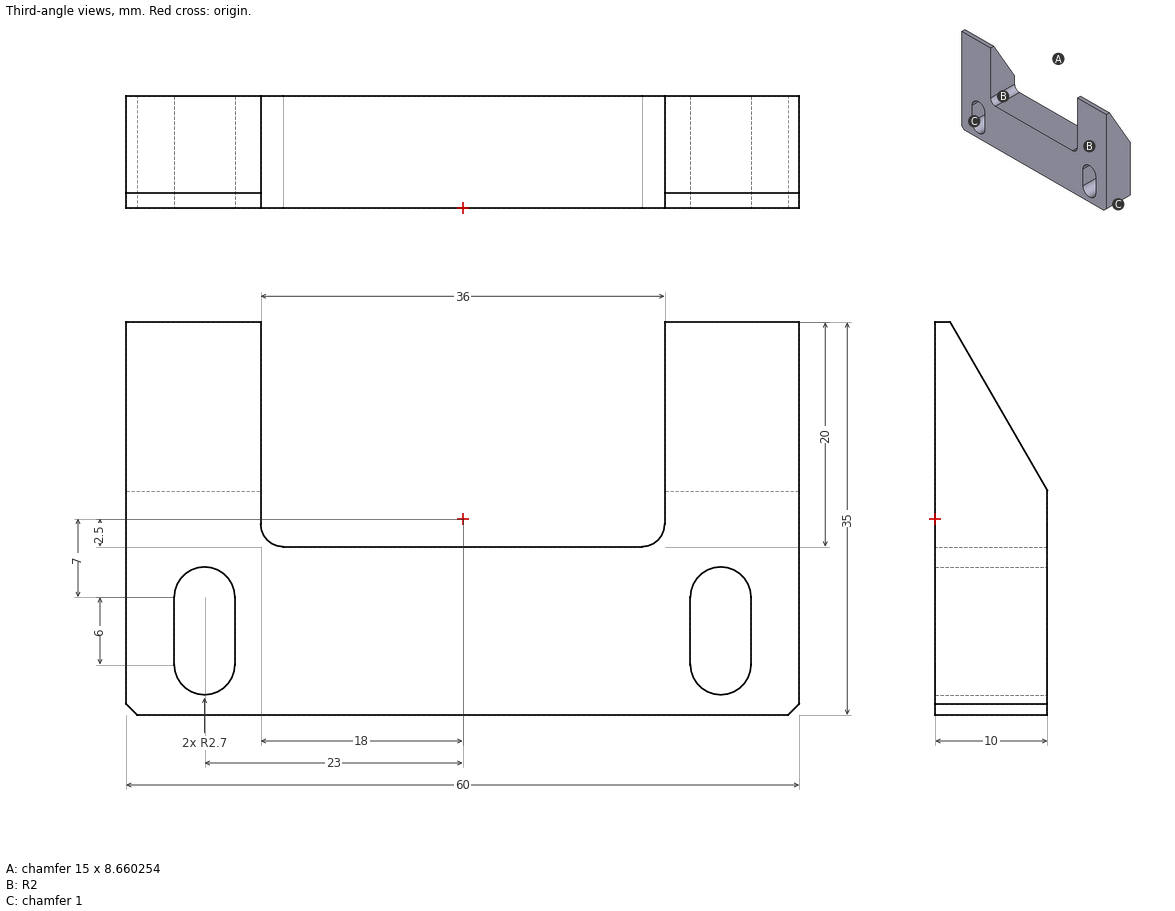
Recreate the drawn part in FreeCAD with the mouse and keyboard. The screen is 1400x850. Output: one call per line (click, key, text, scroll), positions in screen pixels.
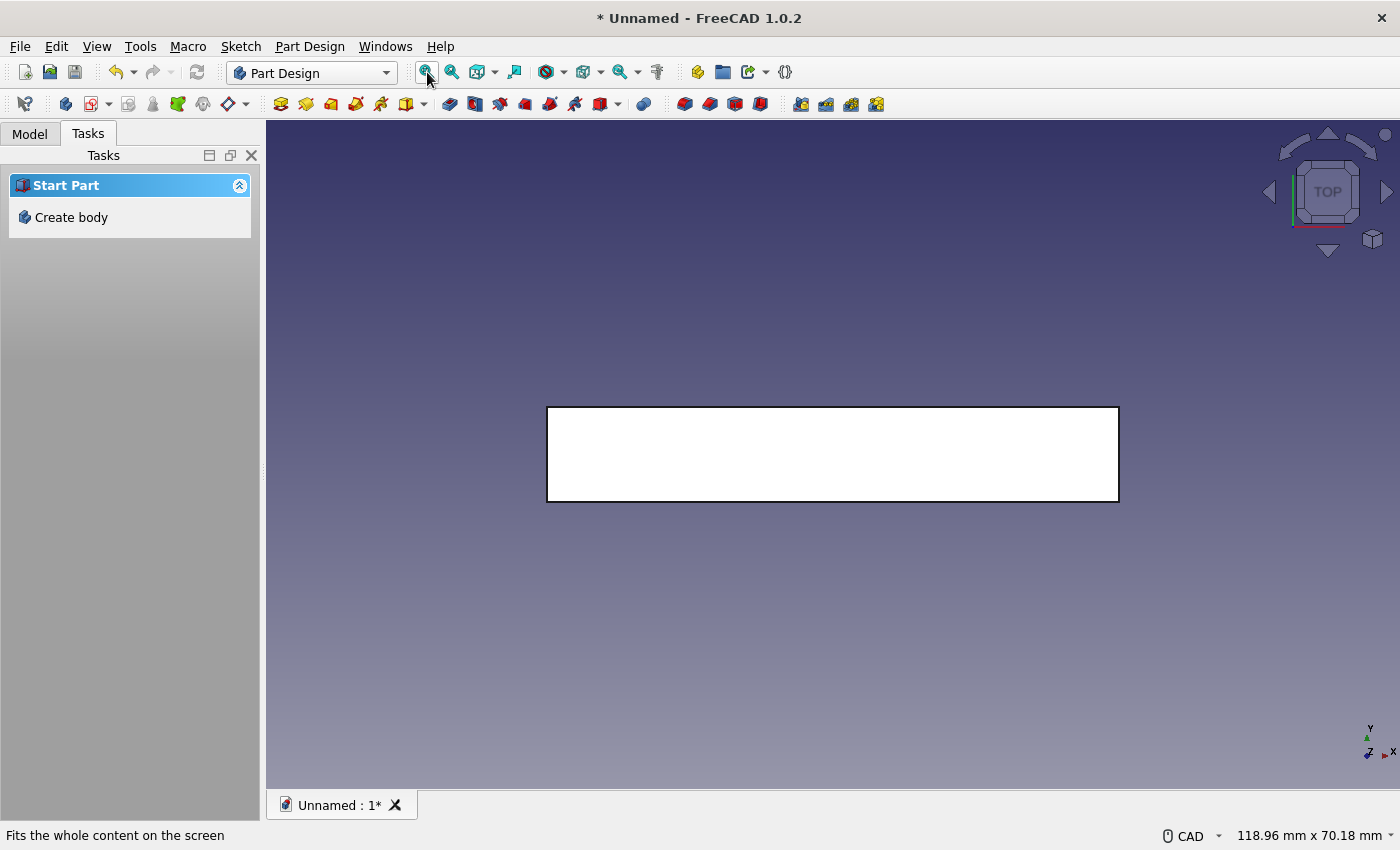
click(833, 406)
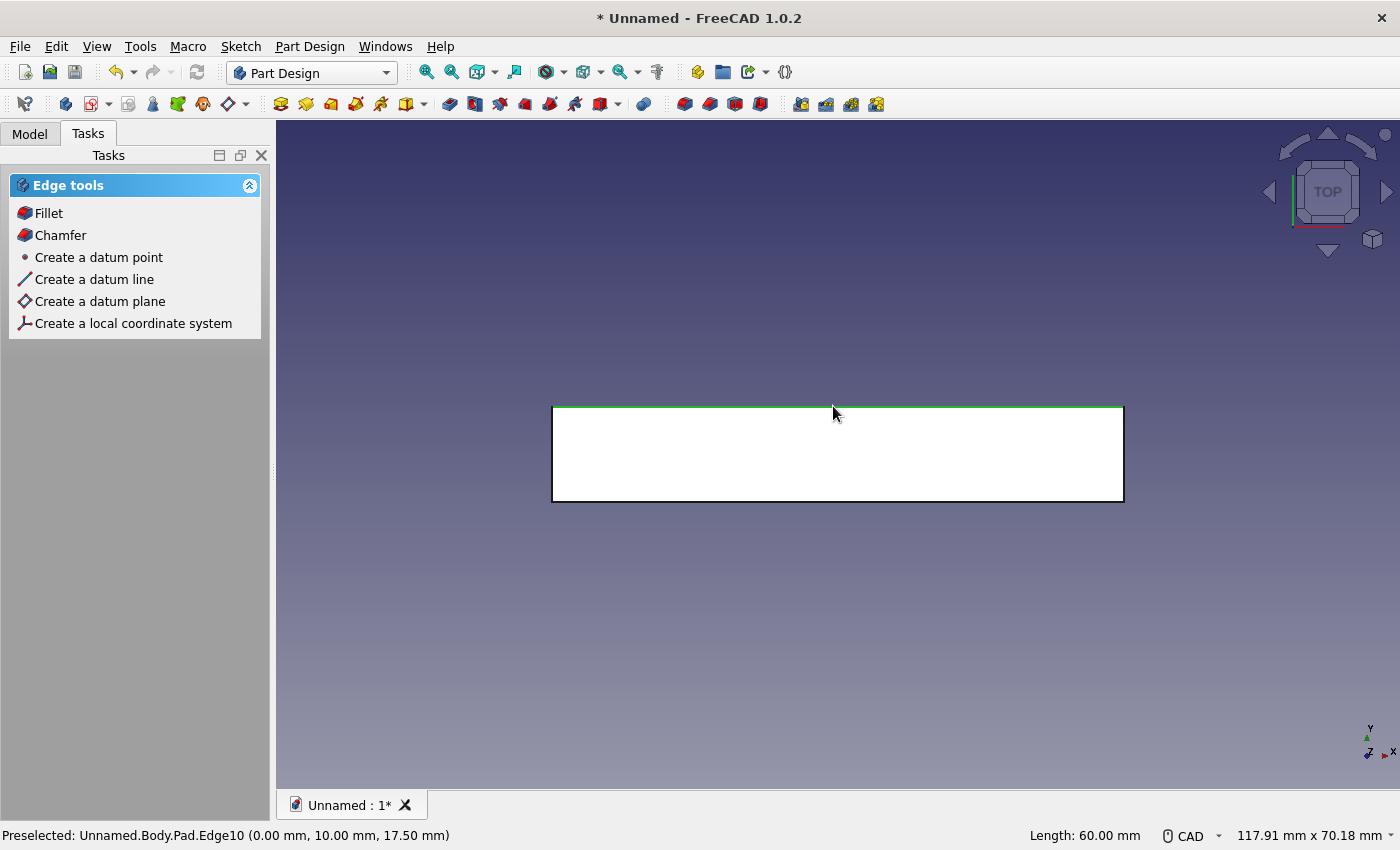
click(710, 104)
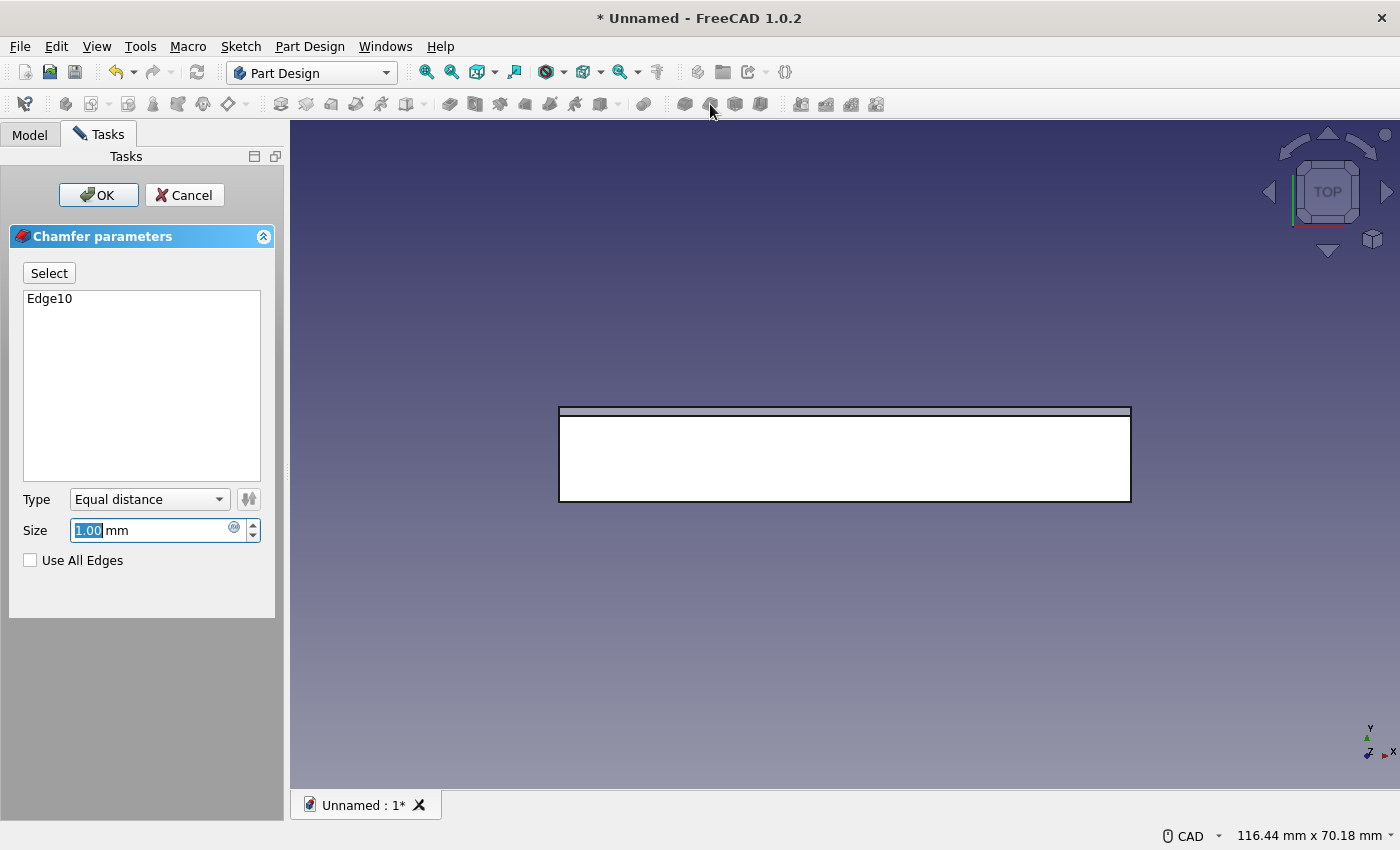
text(15)
key(Tab)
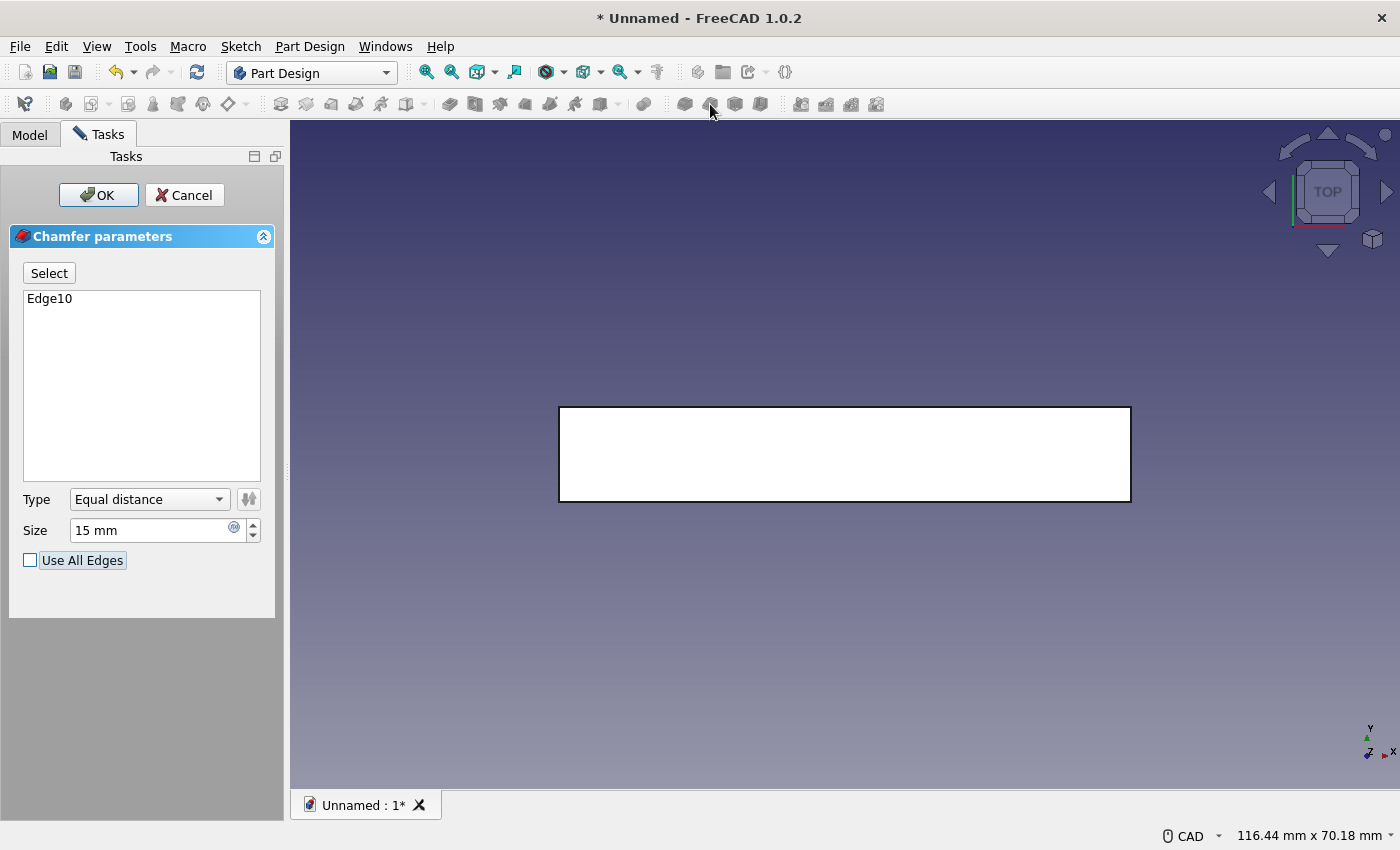
click(150, 500)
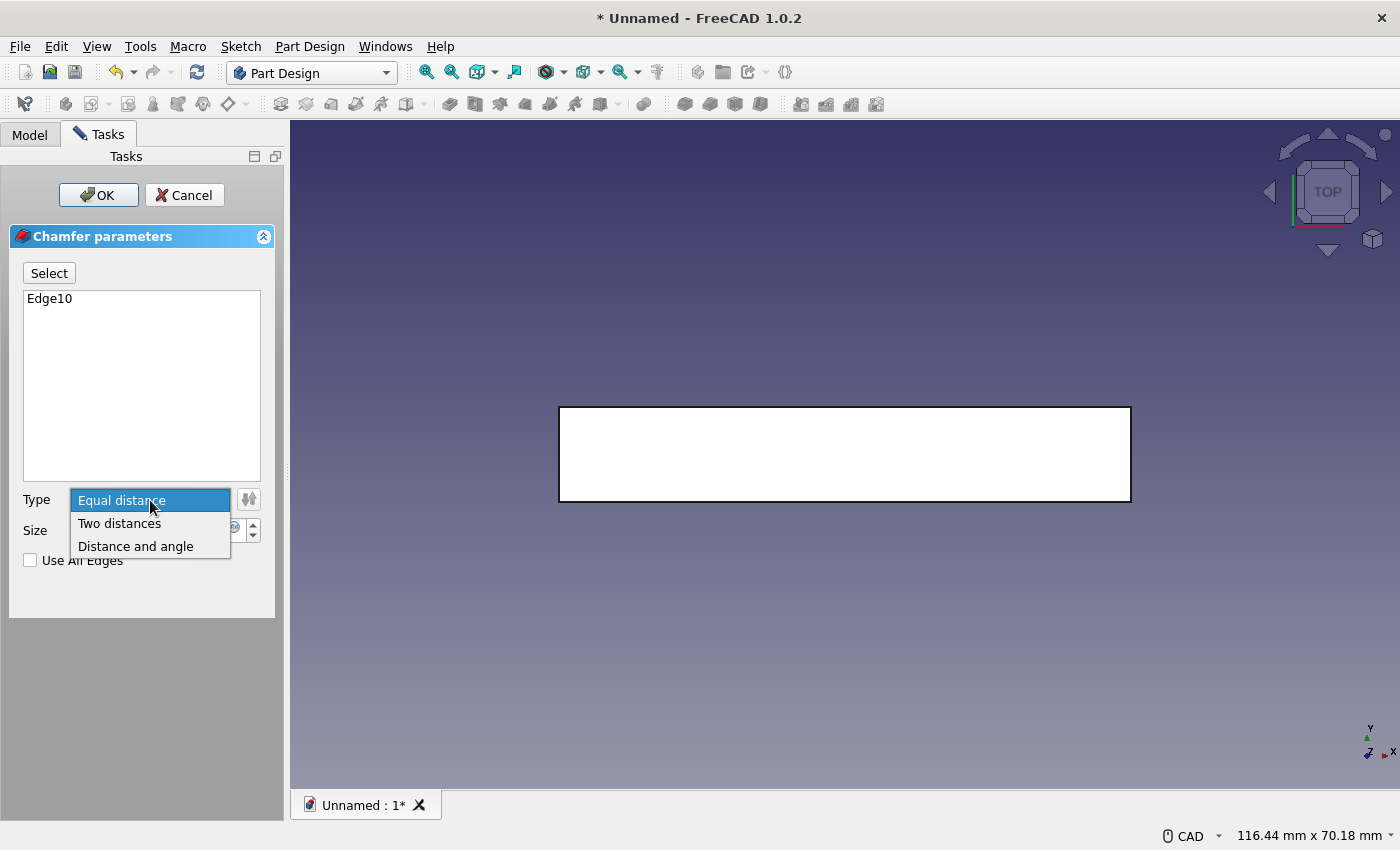
click(148, 524)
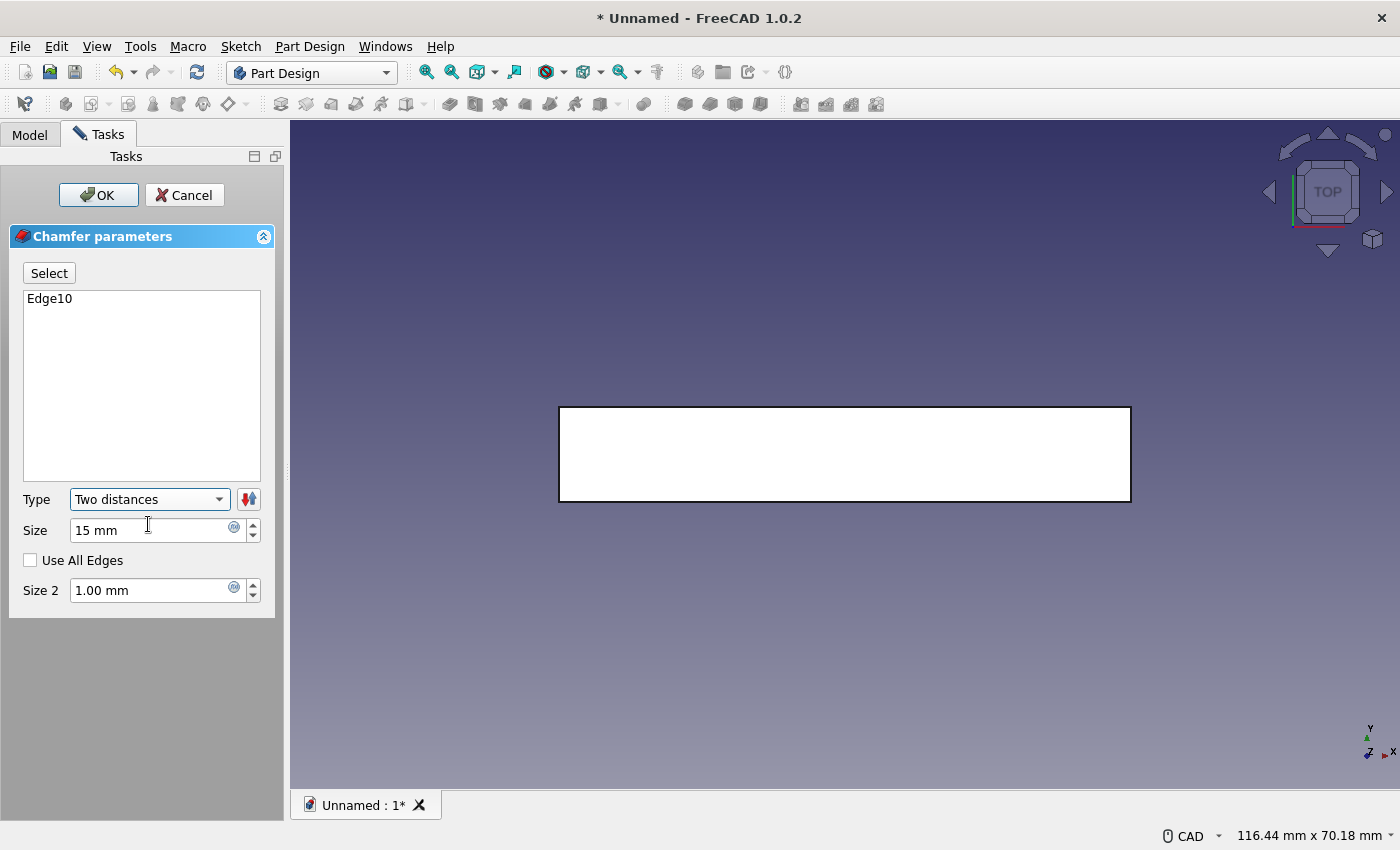
triple_click(158, 590)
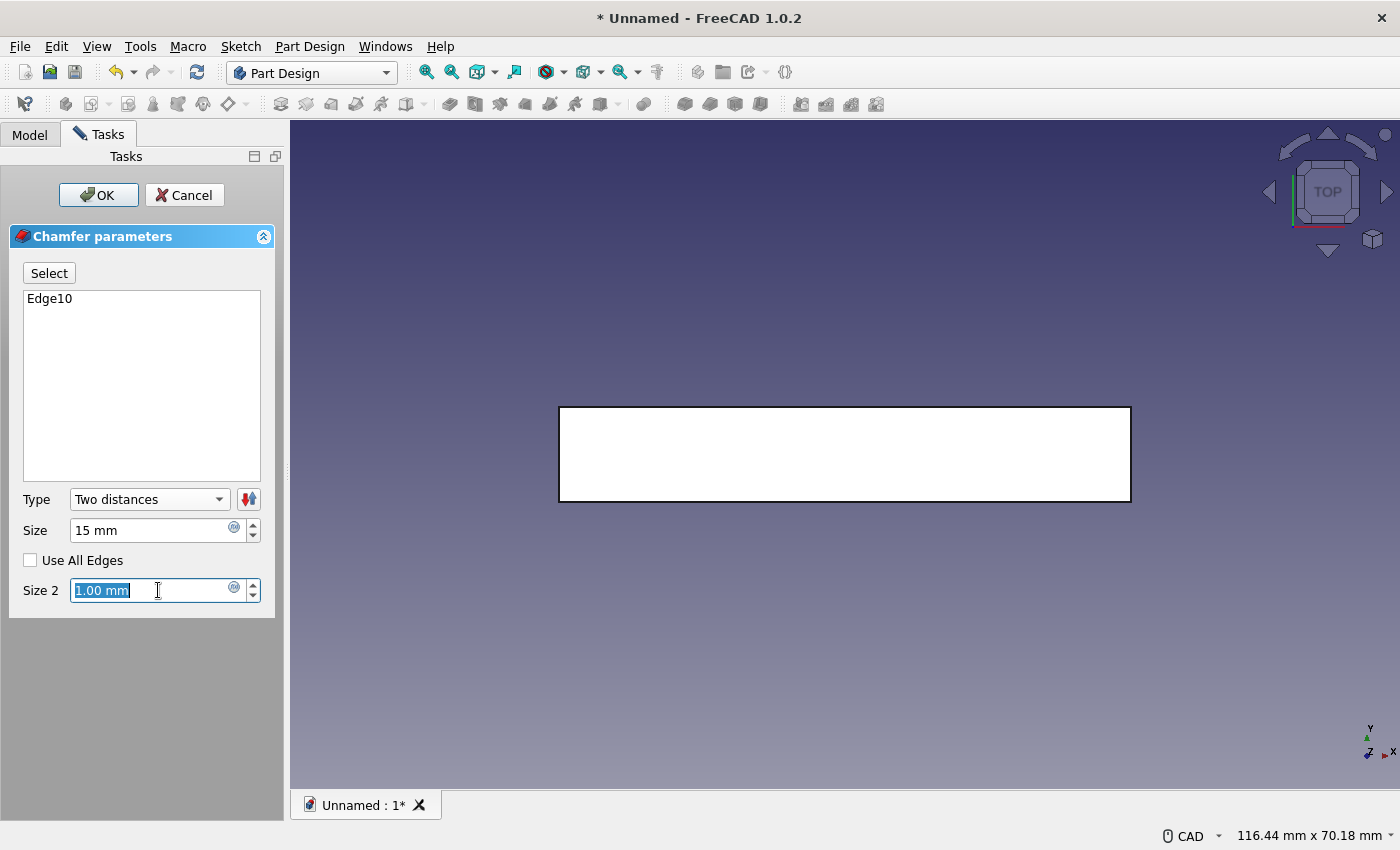
text(8.660254)
key(Tab)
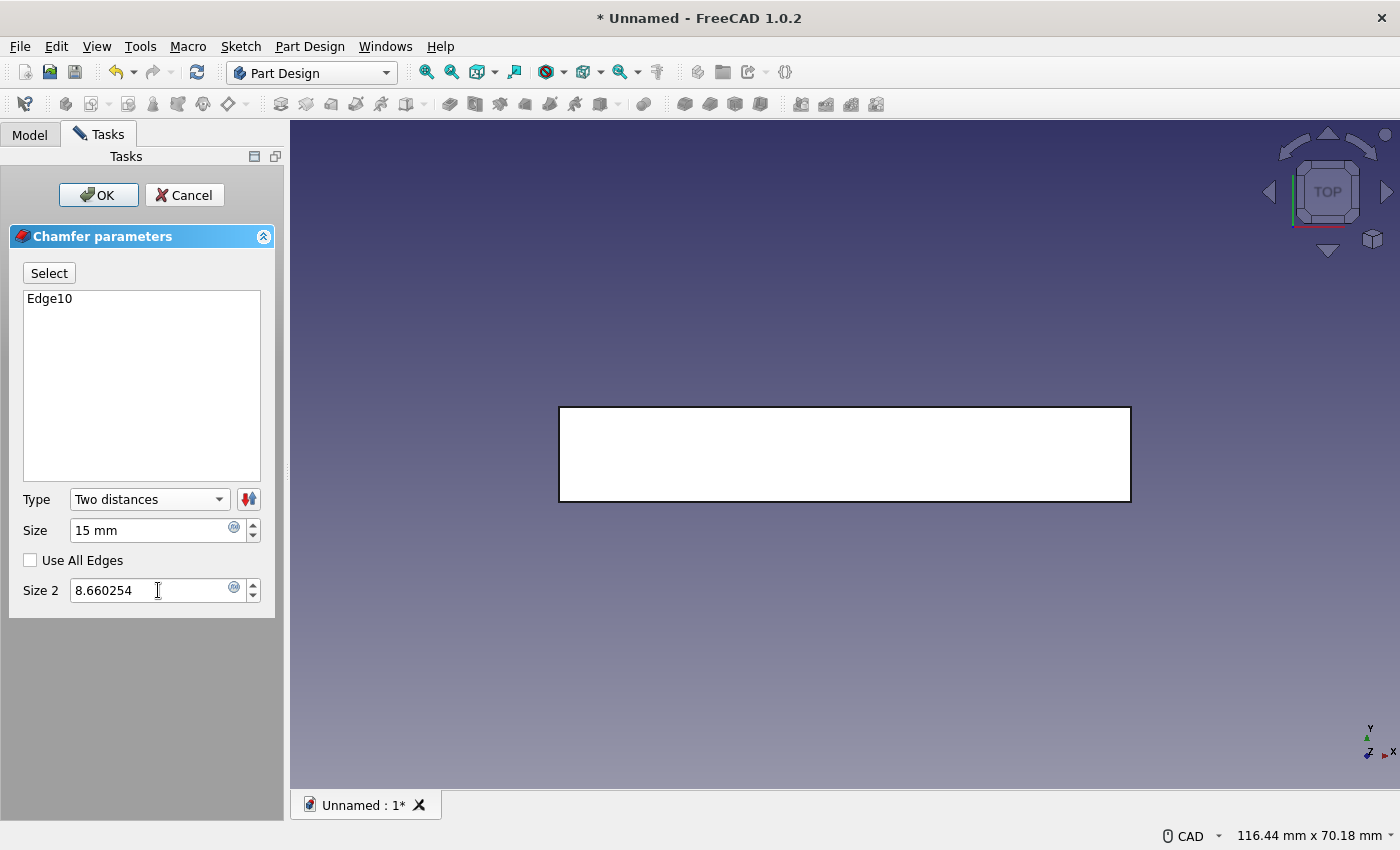
click(249, 500)